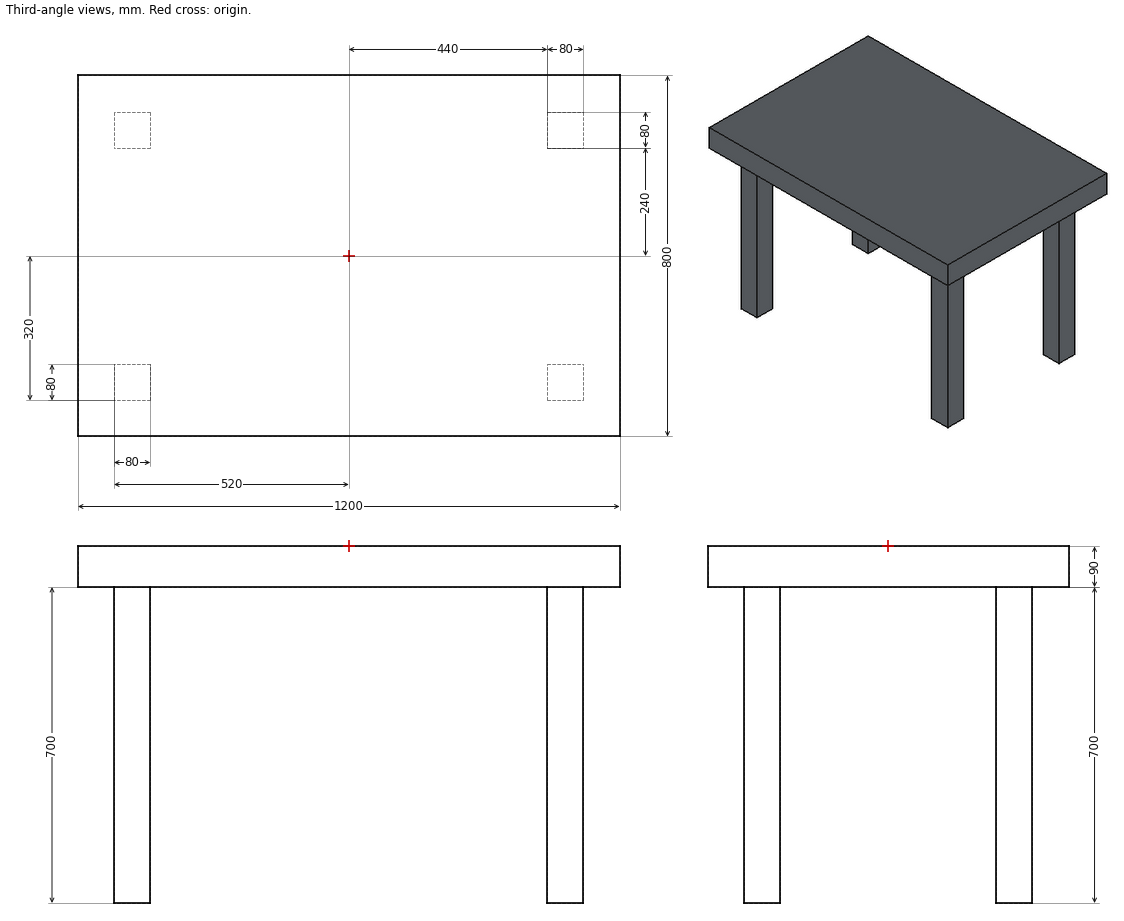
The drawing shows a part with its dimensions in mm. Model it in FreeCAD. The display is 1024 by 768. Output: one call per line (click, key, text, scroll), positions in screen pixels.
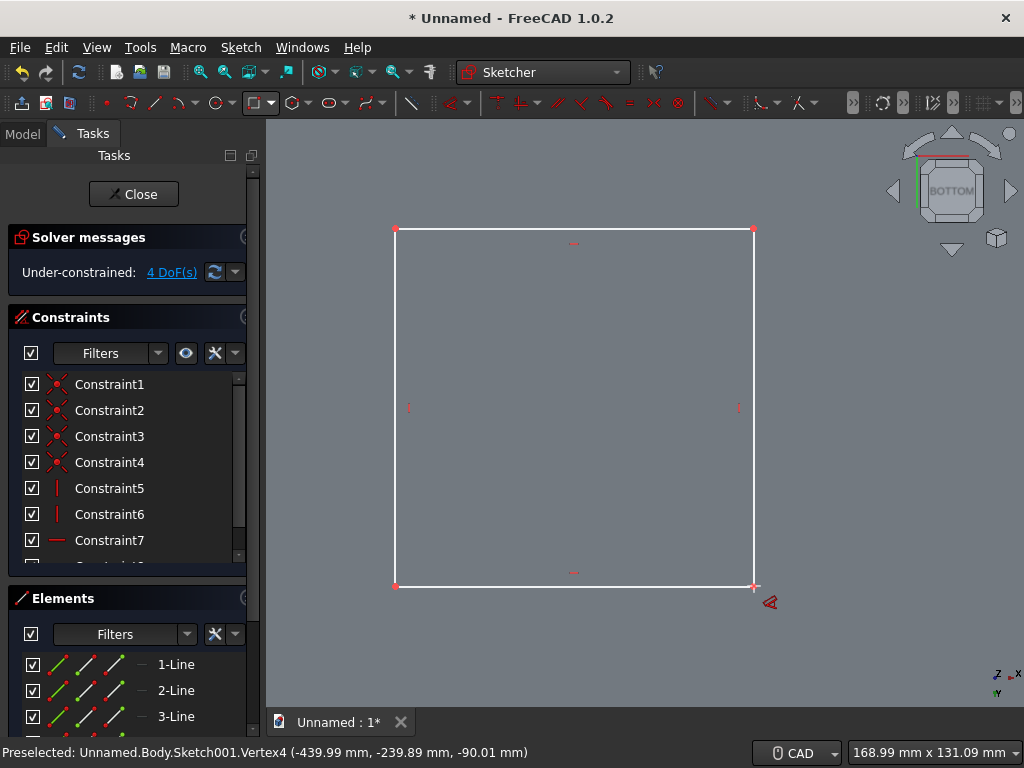
click(395, 336)
click(361, 408)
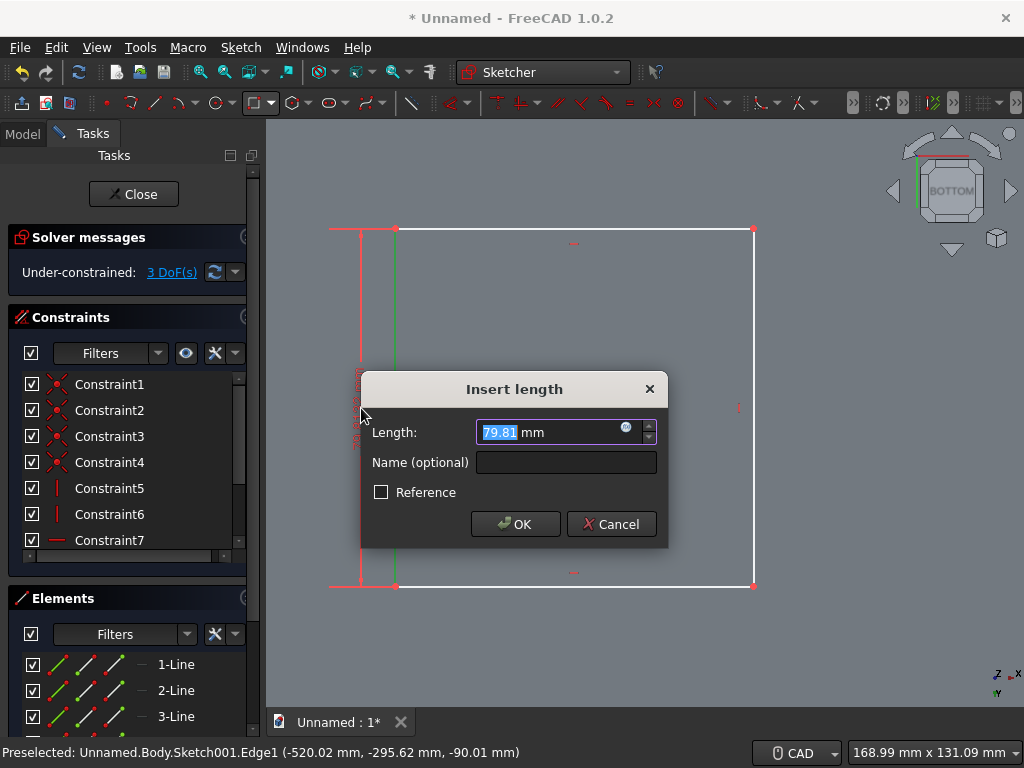
text(80)
key(Return)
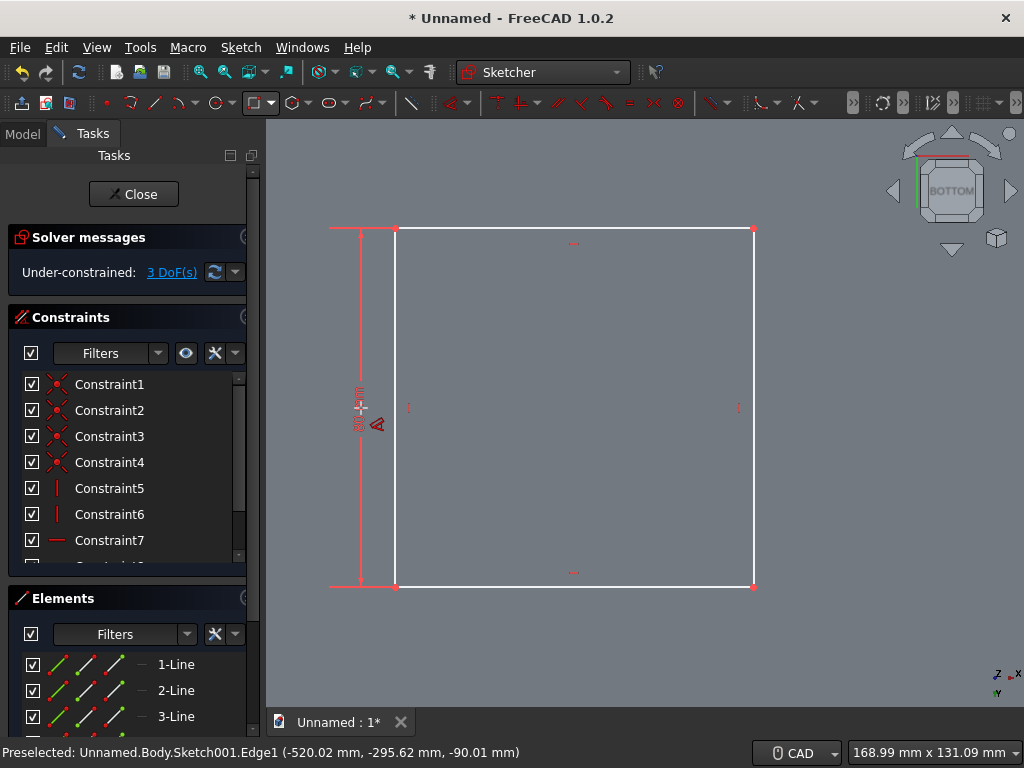
click(503, 587)
click(574, 621)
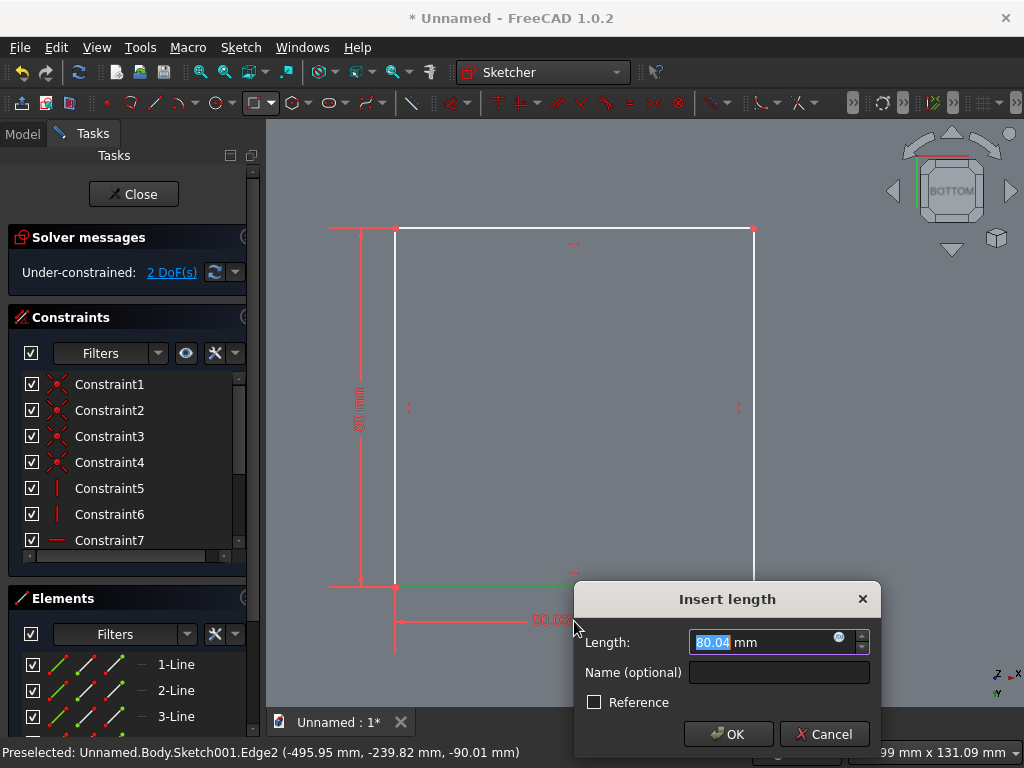
text(80)
key(Return)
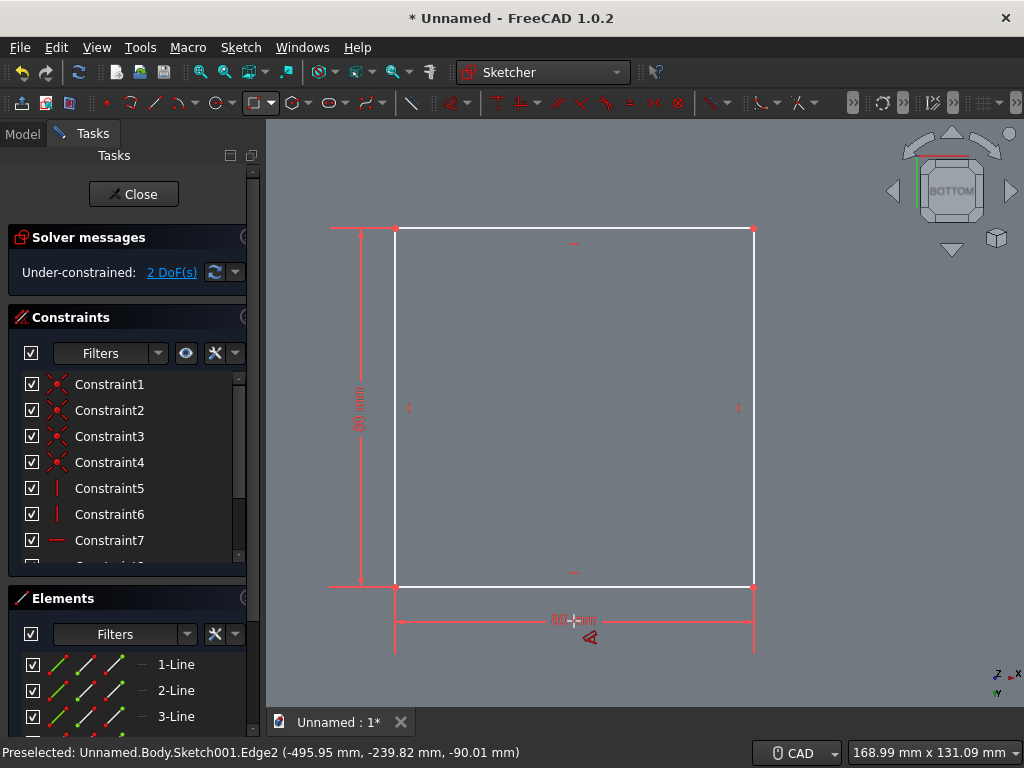
click(395, 228)
click(627, 194)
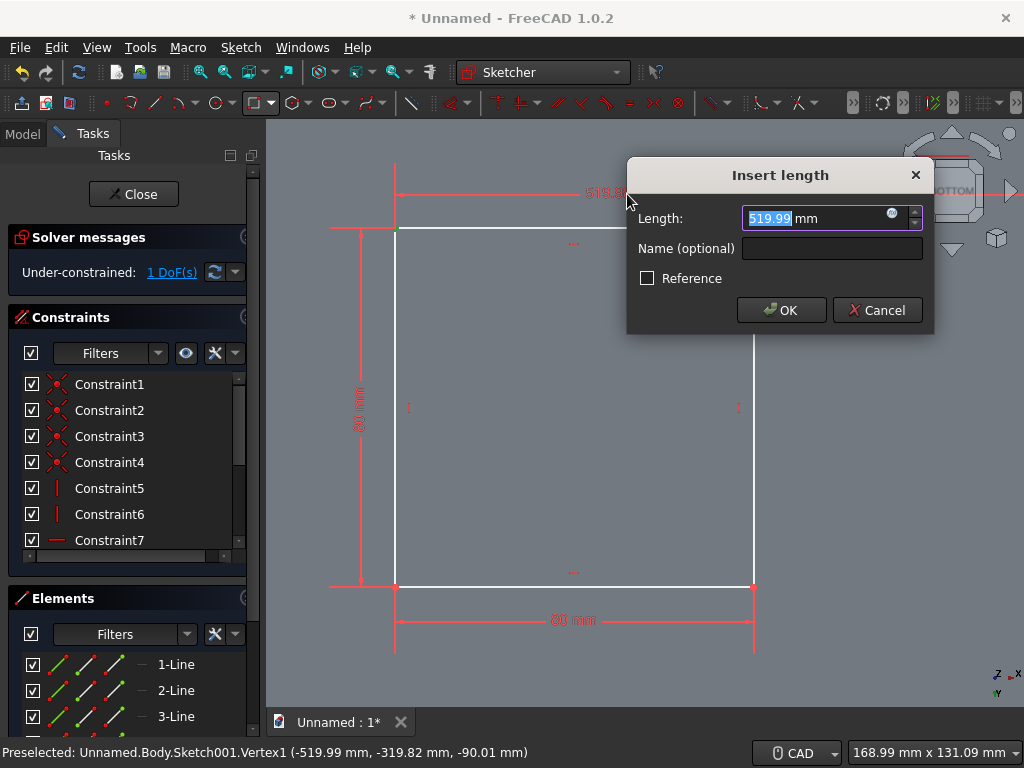
text(520)
key(Return)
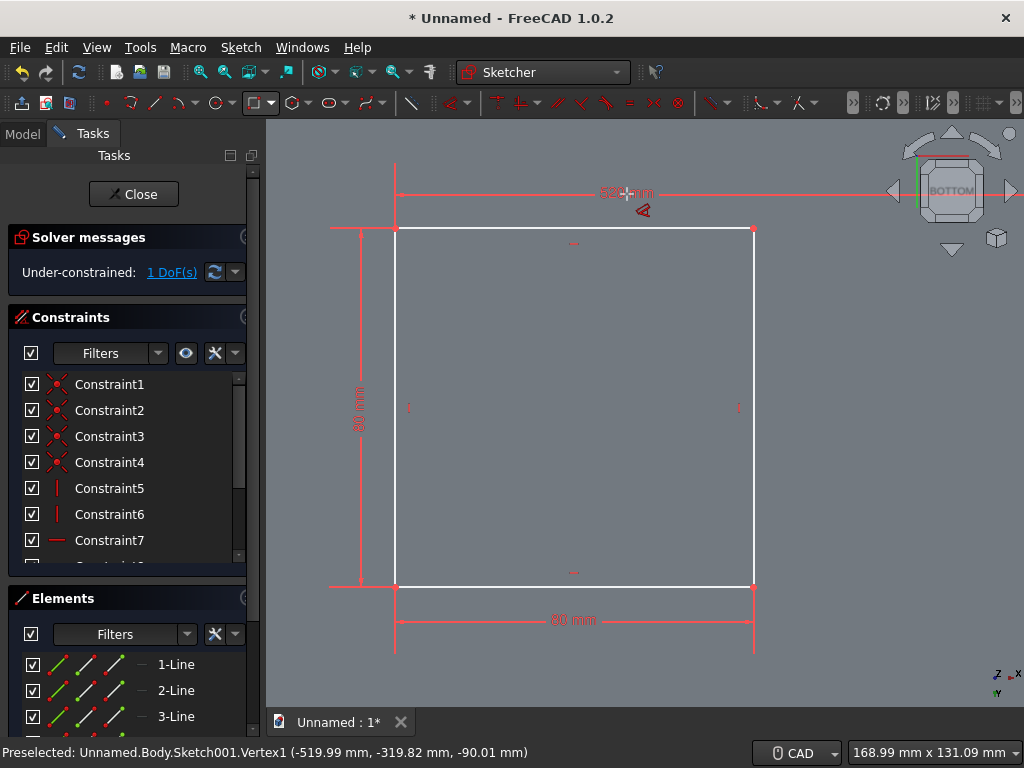
click(395, 228)
click(361, 454)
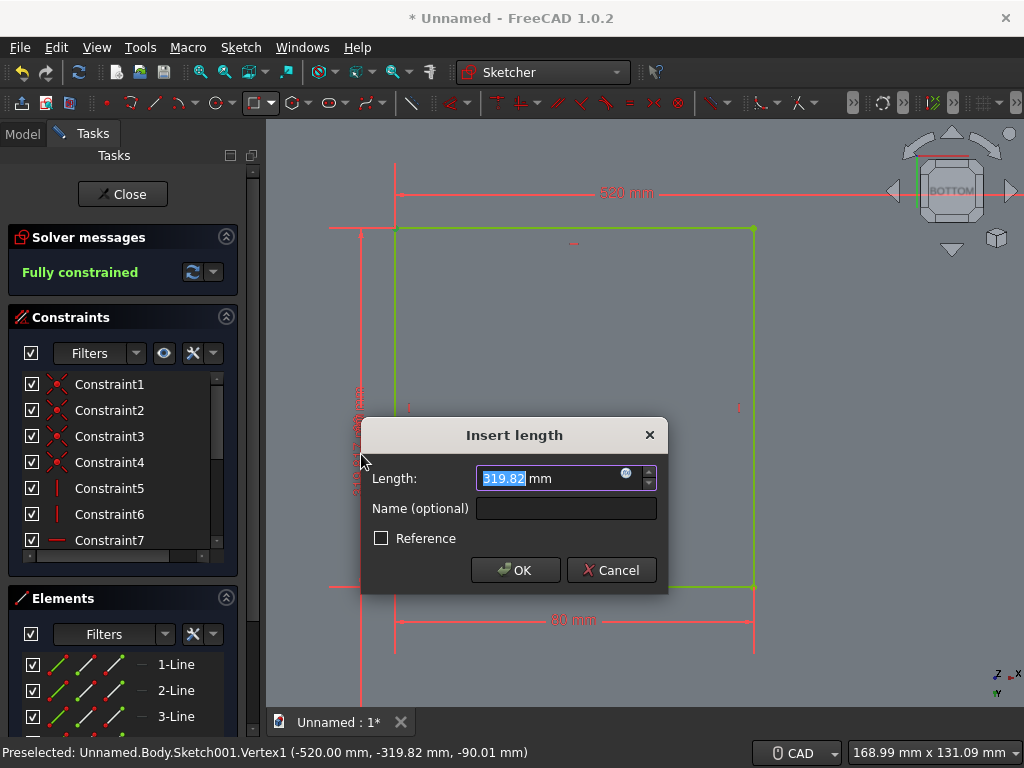
text(320)
key(Return)
key(Escape)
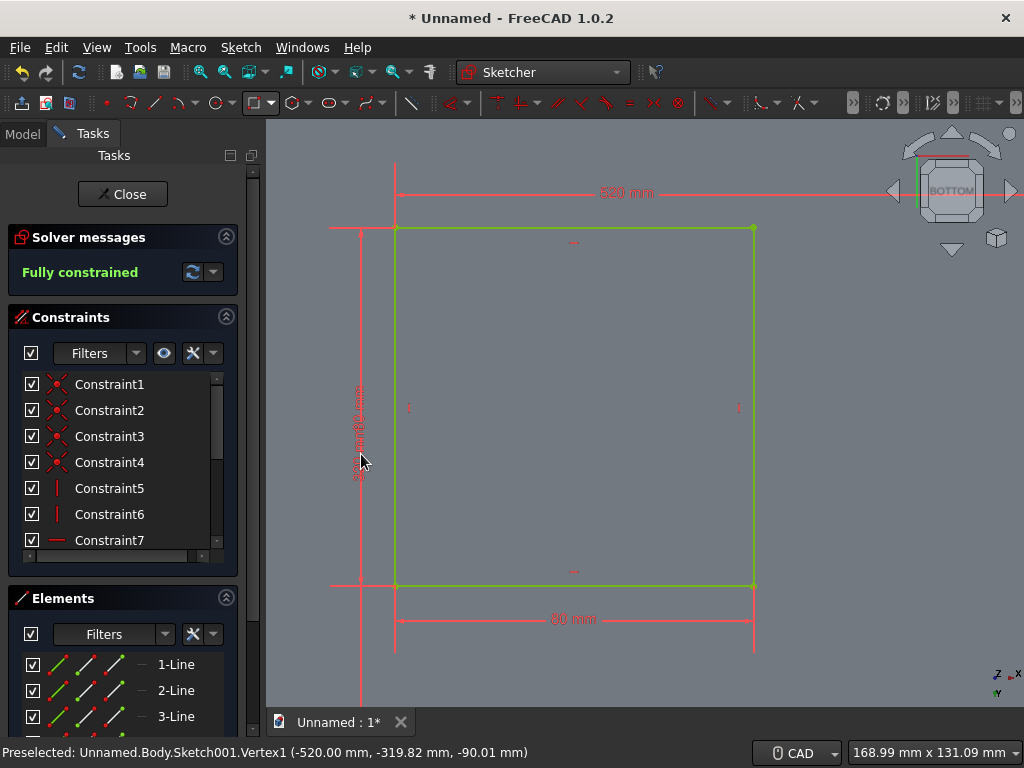
click(123, 194)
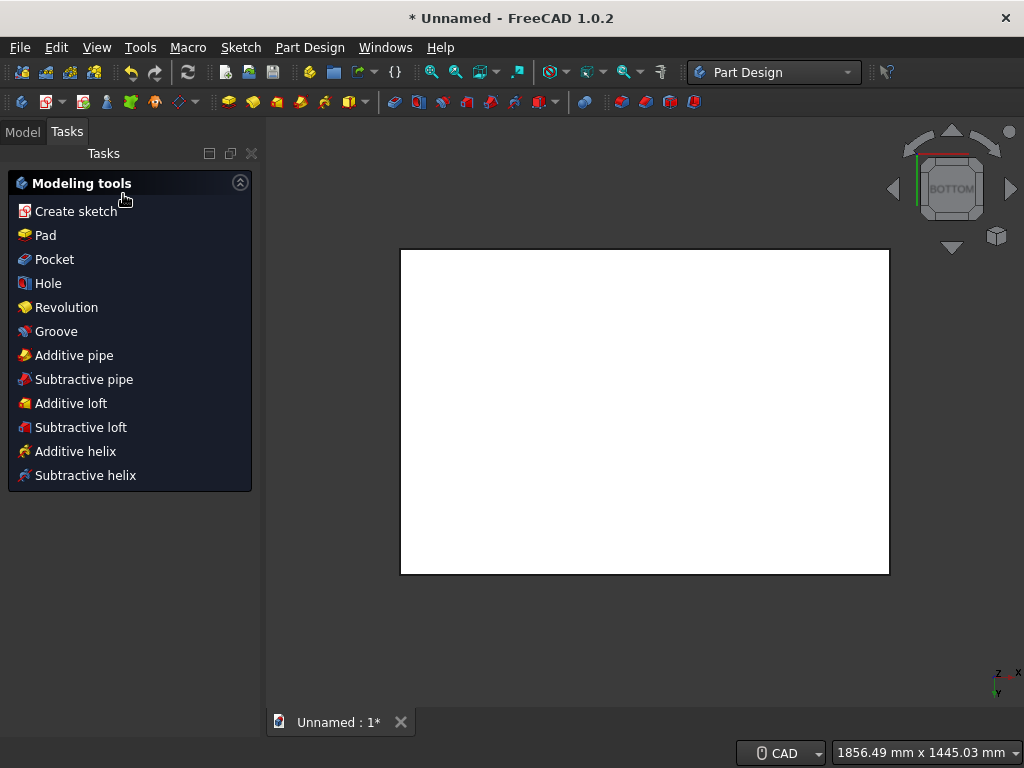
click(230, 102)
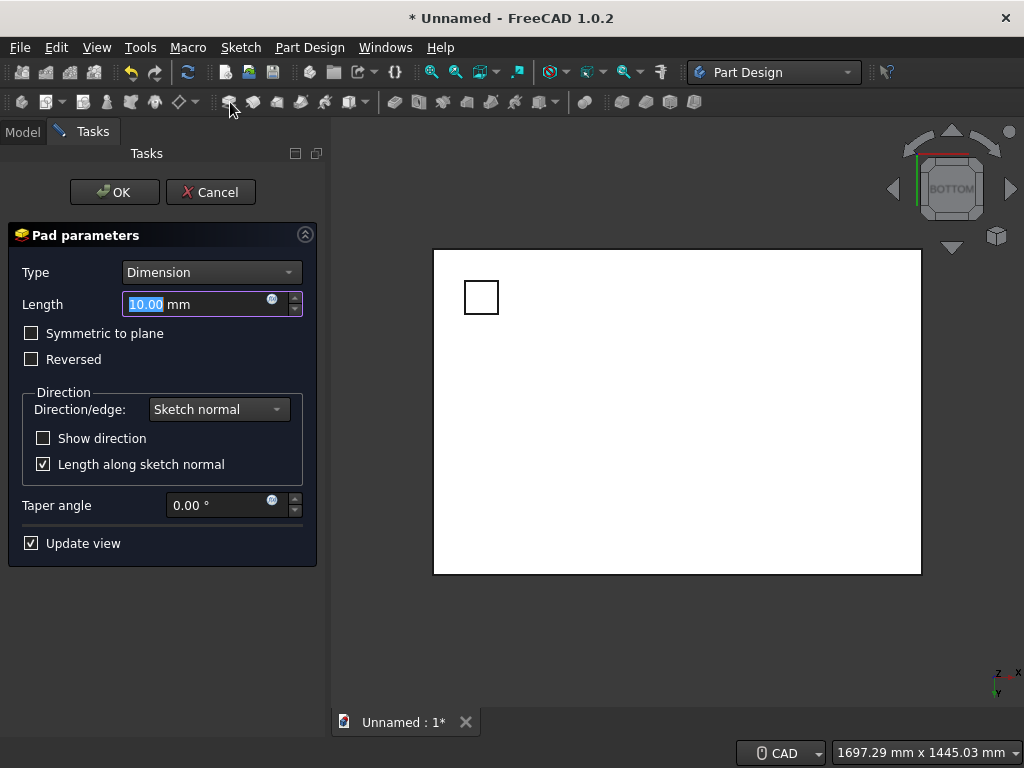
text(700)
key(Tab)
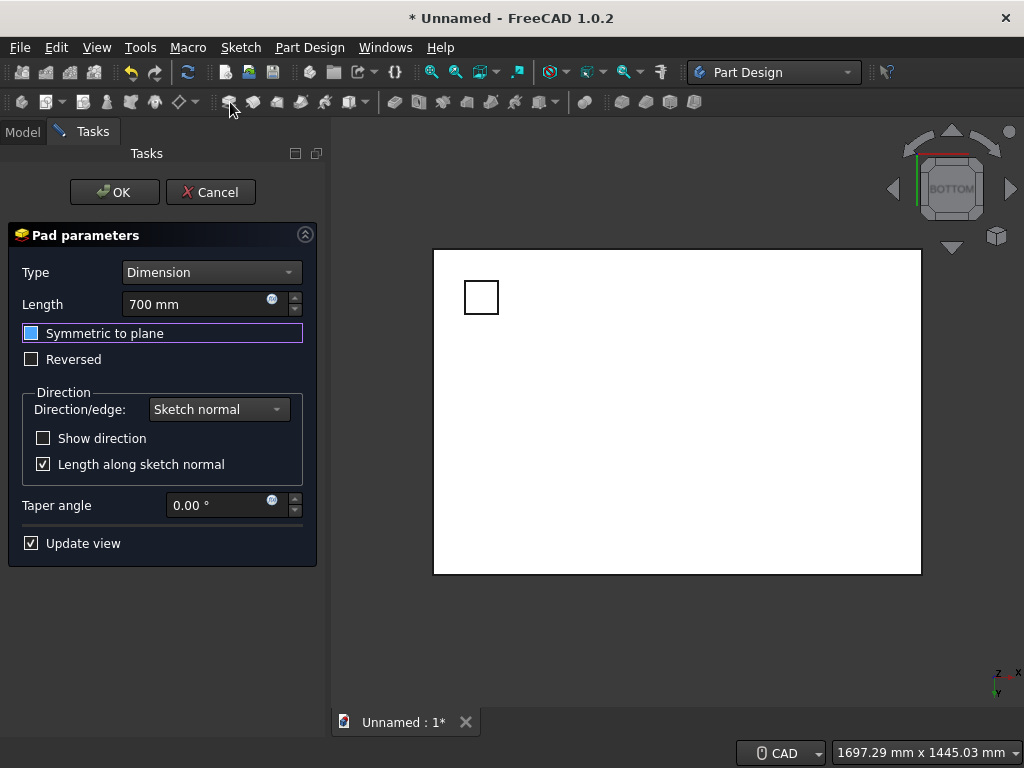
click(115, 192)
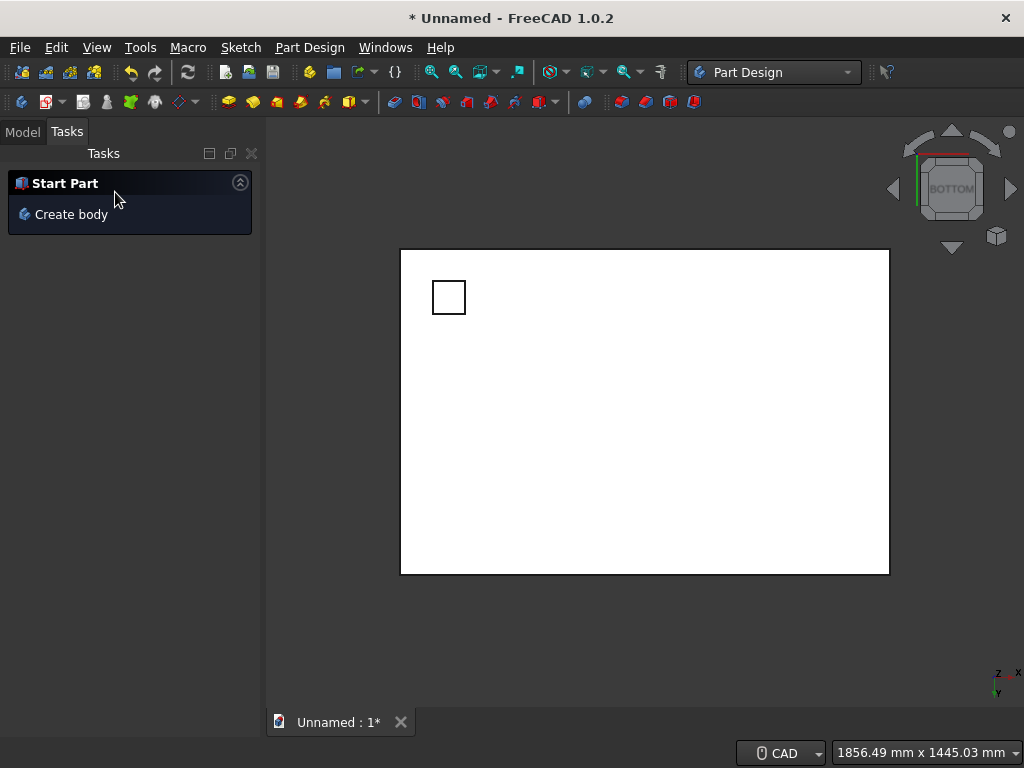
click(23, 131)